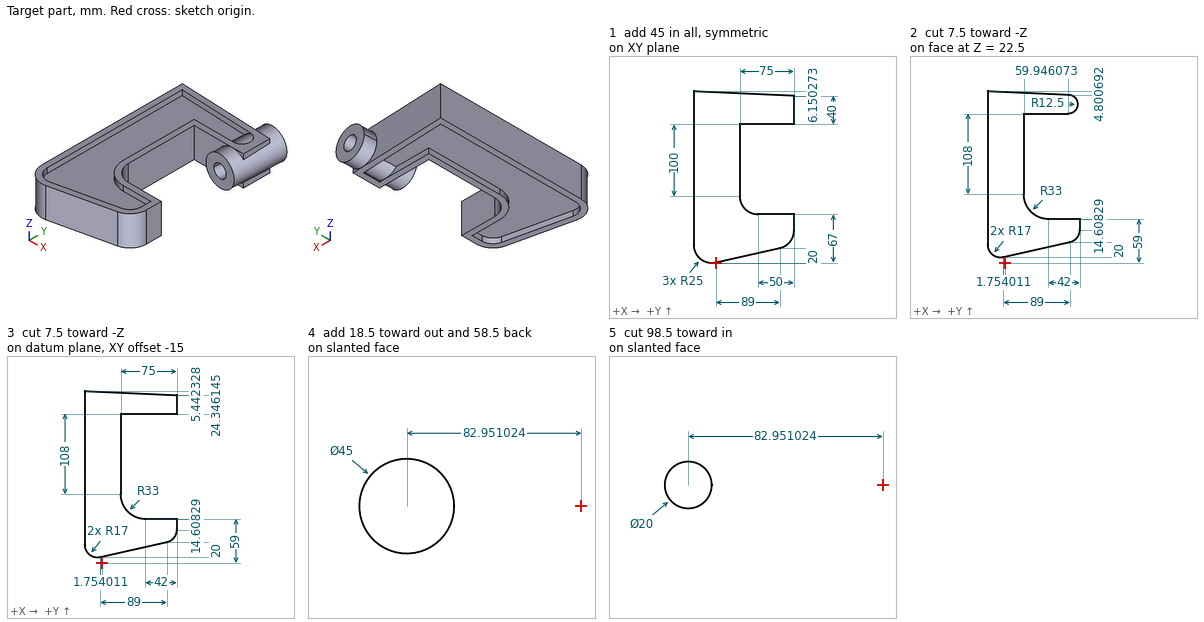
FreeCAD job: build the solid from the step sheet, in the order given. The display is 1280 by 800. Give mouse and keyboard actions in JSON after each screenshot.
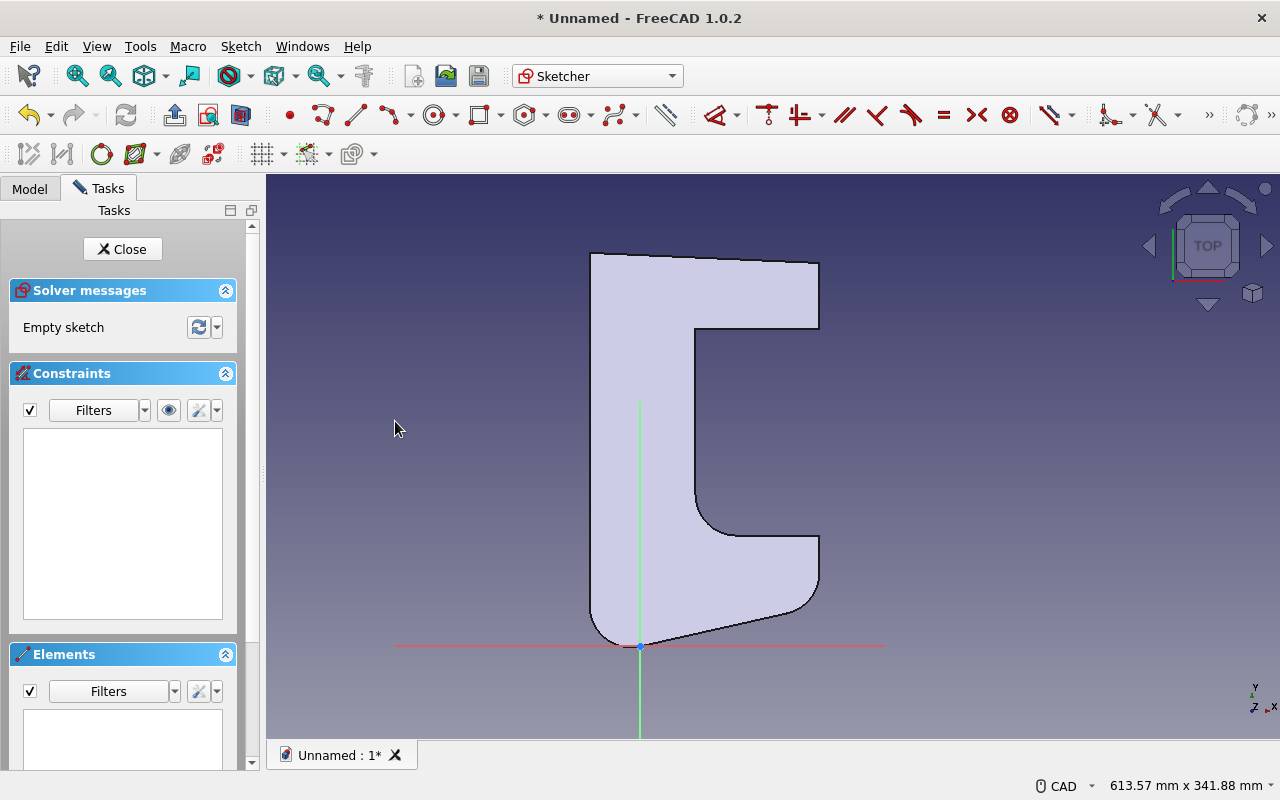
{"action": "left_click", "coordinate": [356, 116]}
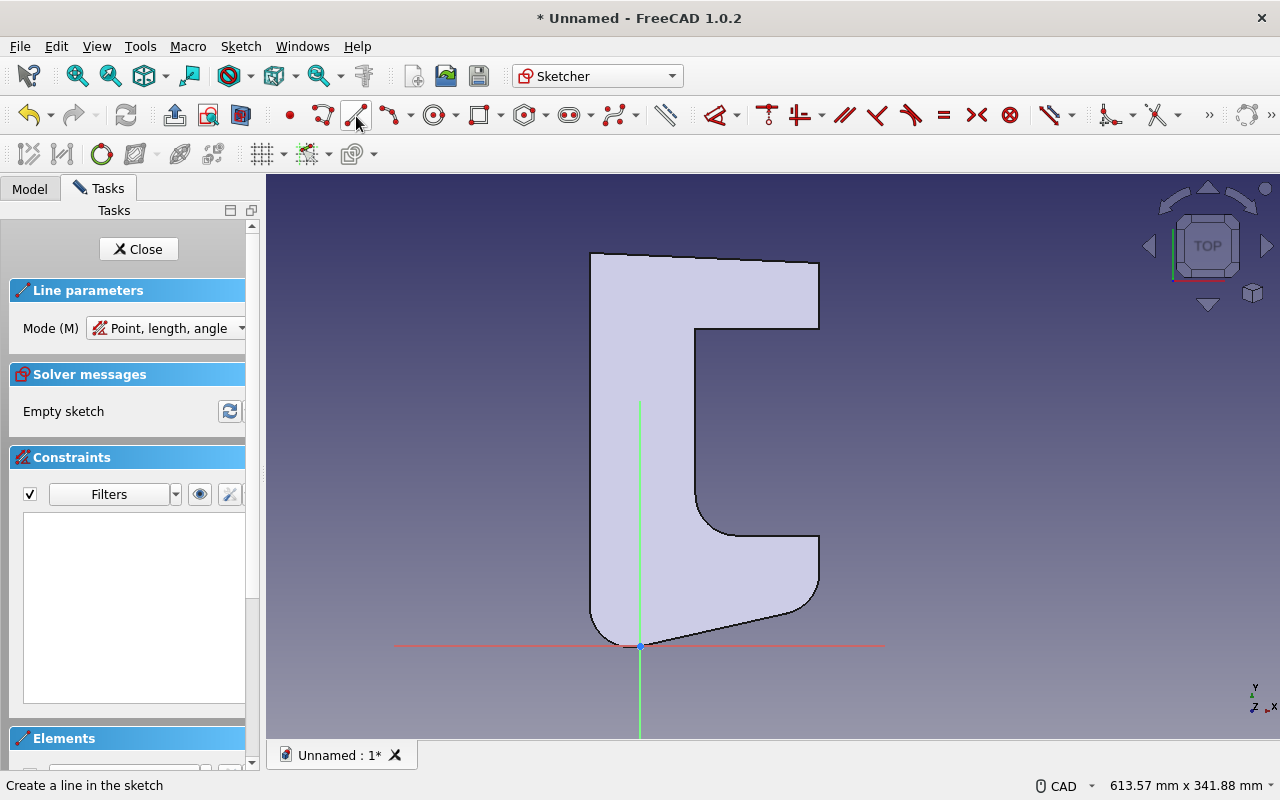
{"action": "scroll", "coordinate": [637, 634], "scroll_direction": "up", "scroll_amount": 9}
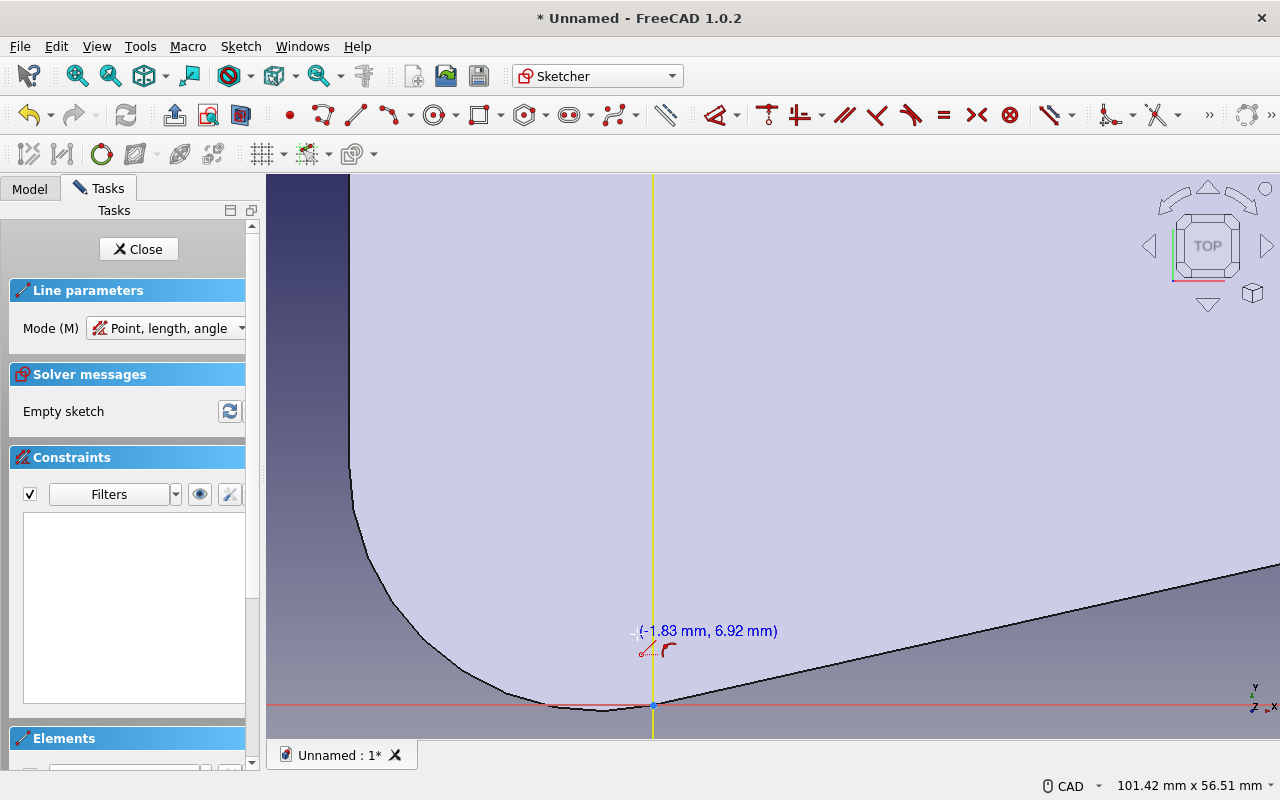
{"action": "left_click", "coordinate": [636, 627]}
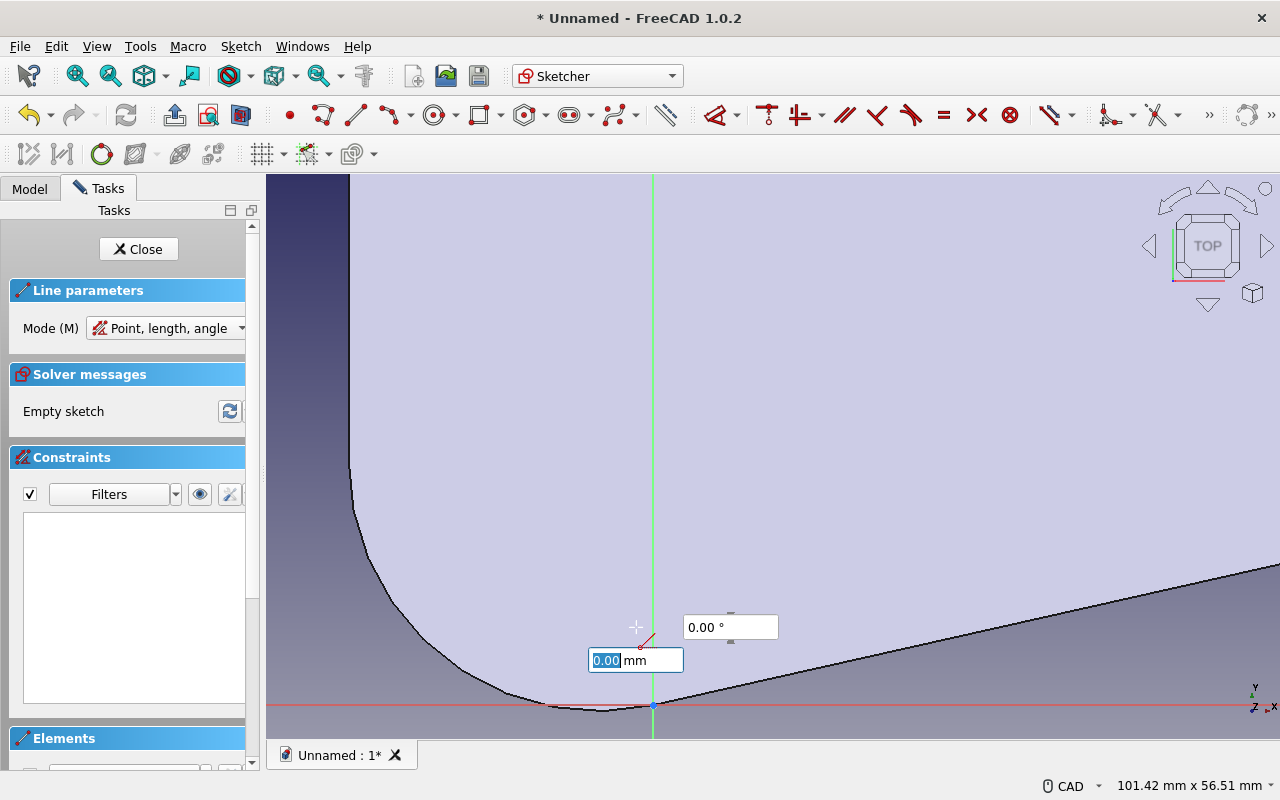
{"action": "scroll", "coordinate": [637, 635], "scroll_direction": "down", "scroll_amount": 9}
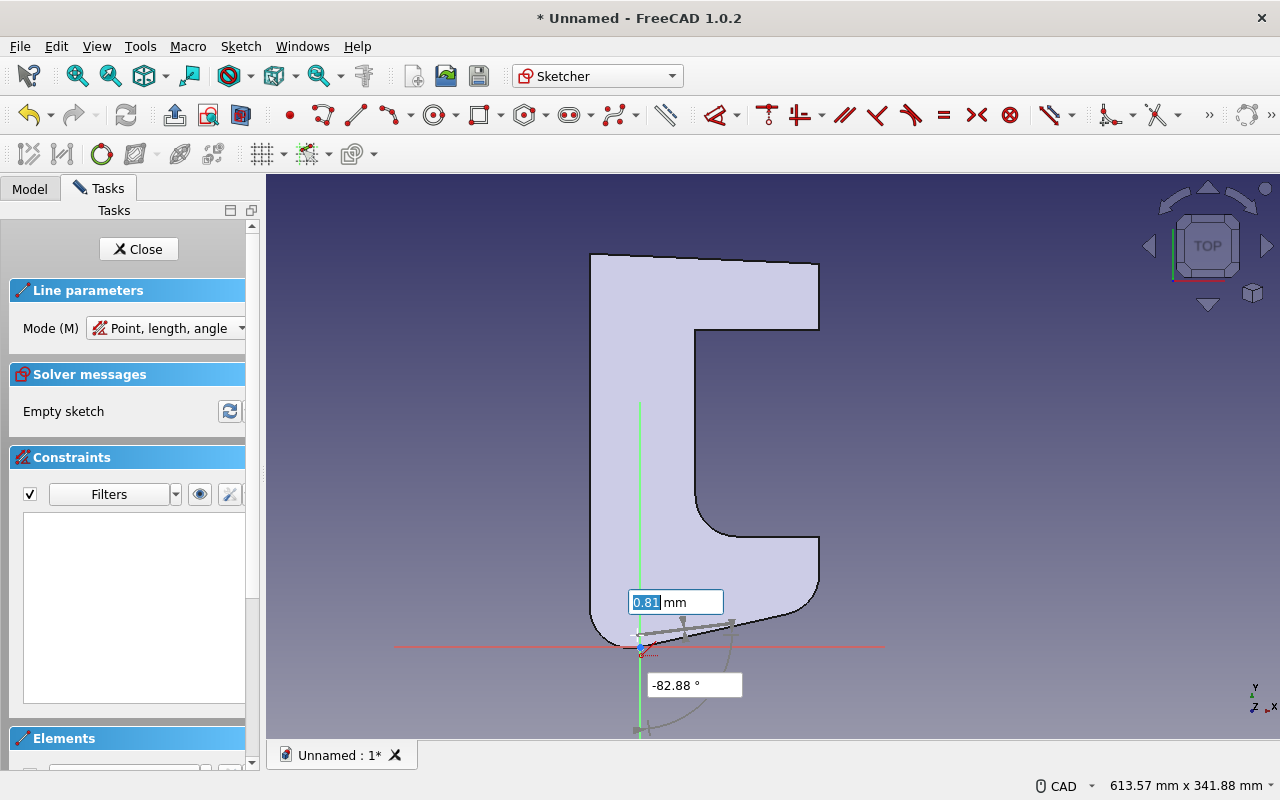
{"action": "left_click", "coordinate": [784, 601]}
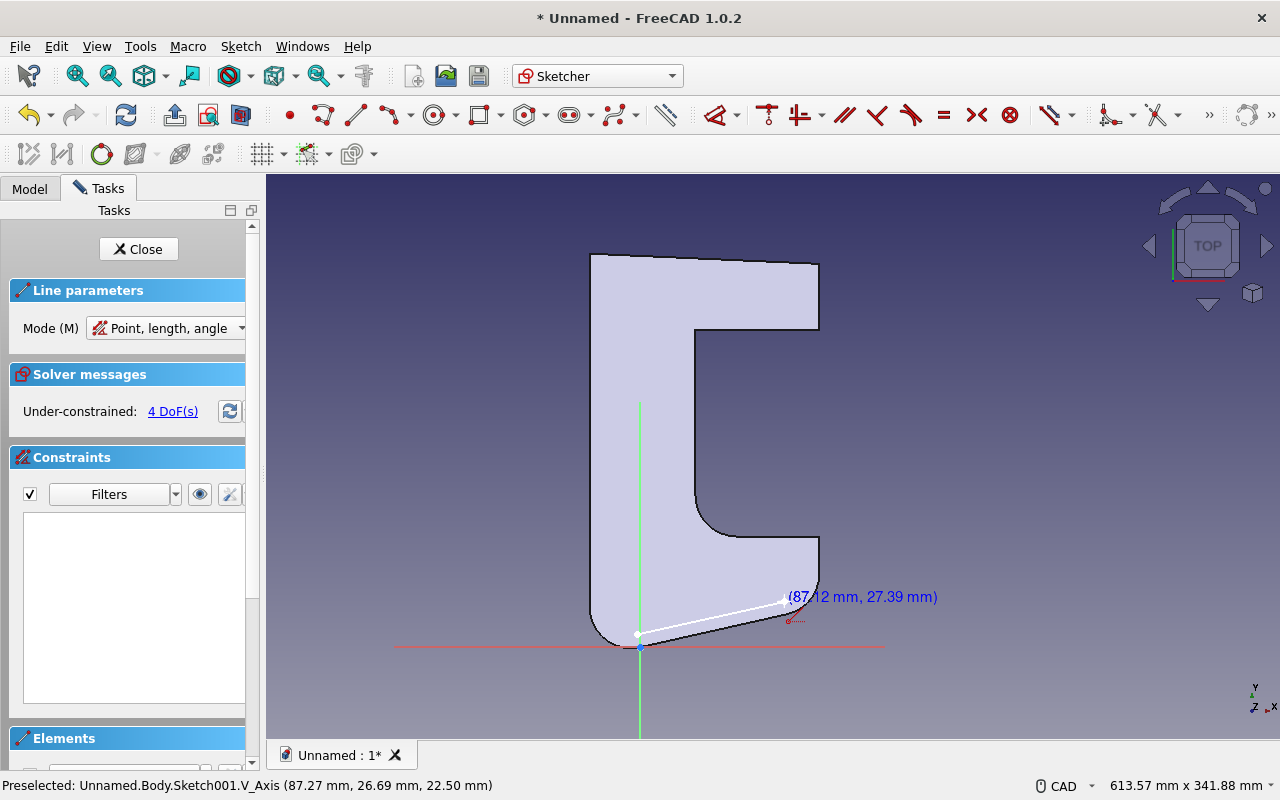
{"action": "left_click", "coordinate": [323, 116]}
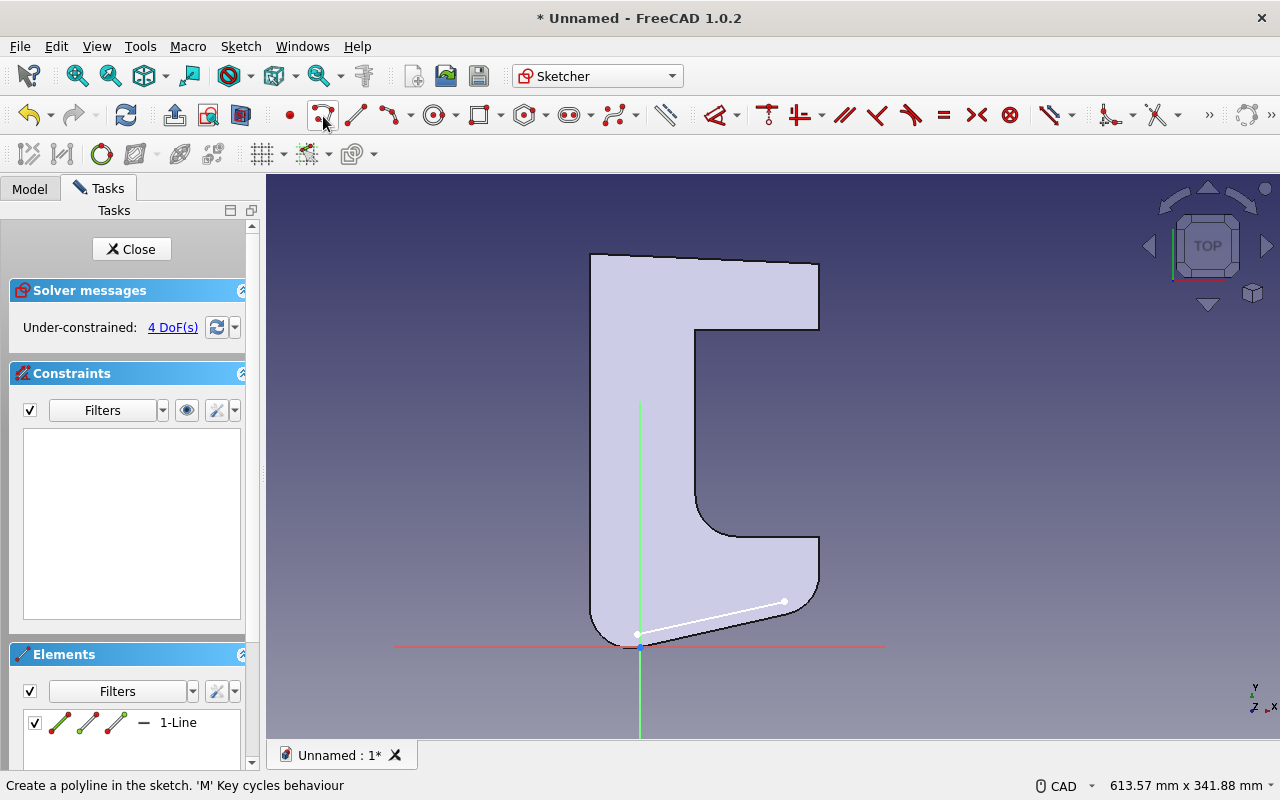
{"action": "left_click", "coordinate": [806, 574]}
{"action": "left_click", "coordinate": [806, 550]}
{"action": "left_click", "coordinate": [737, 550]}
{"action": "right_click", "coordinate": [737, 550]}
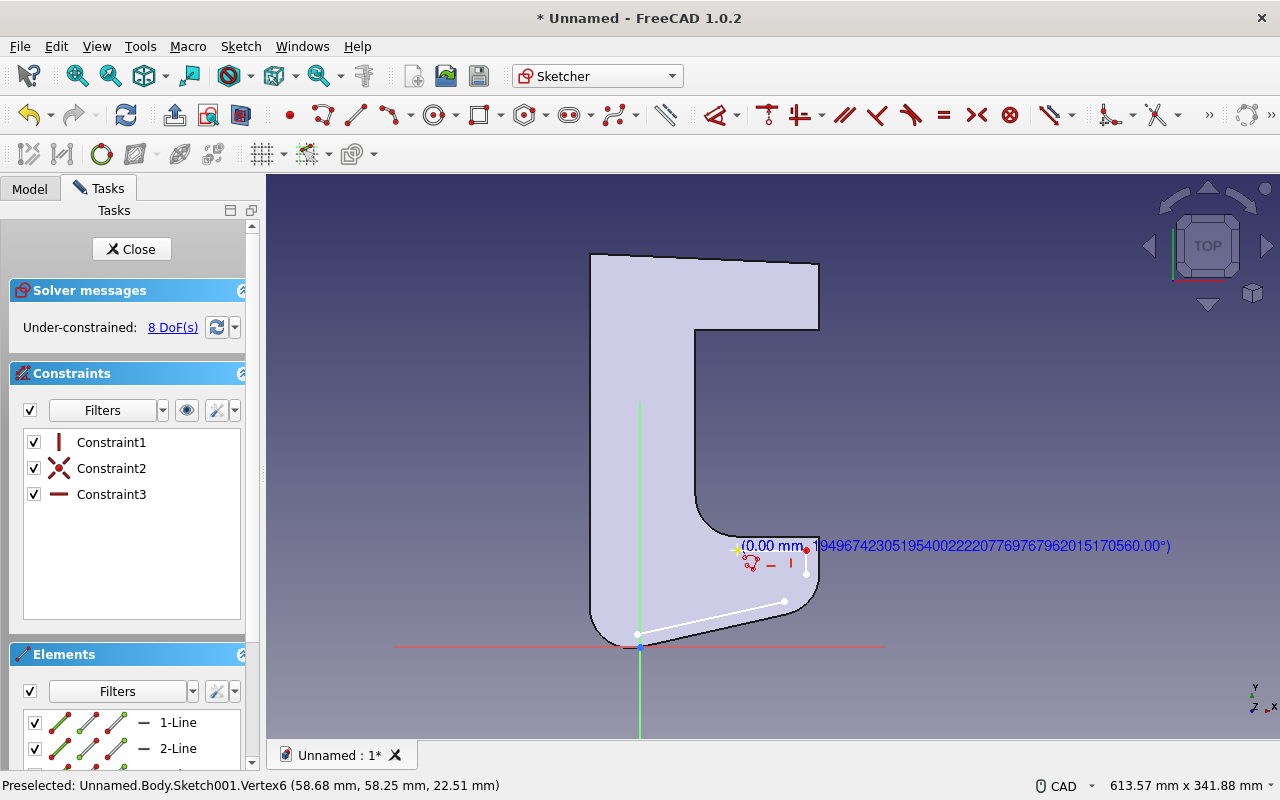
{"action": "left_click", "coordinate": [682, 495]}
{"action": "left_click", "coordinate": [682, 317]}
{"action": "left_click", "coordinate": [781, 317]}
{"action": "right_click", "coordinate": [781, 317]}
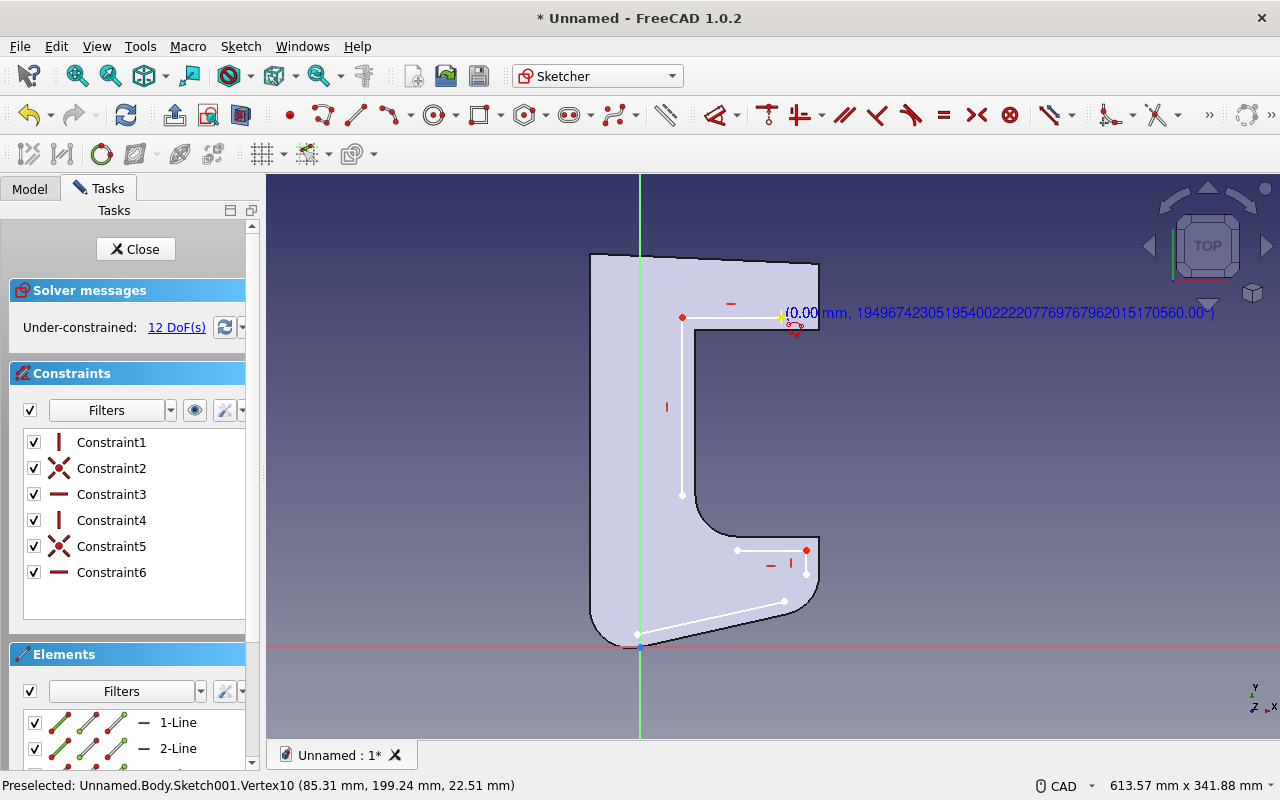
{"action": "left_click", "coordinate": [782, 275]}
{"action": "left_click", "coordinate": [603, 265]}
{"action": "left_click", "coordinate": [603, 607]}
{"action": "right_click", "coordinate": [603, 607]}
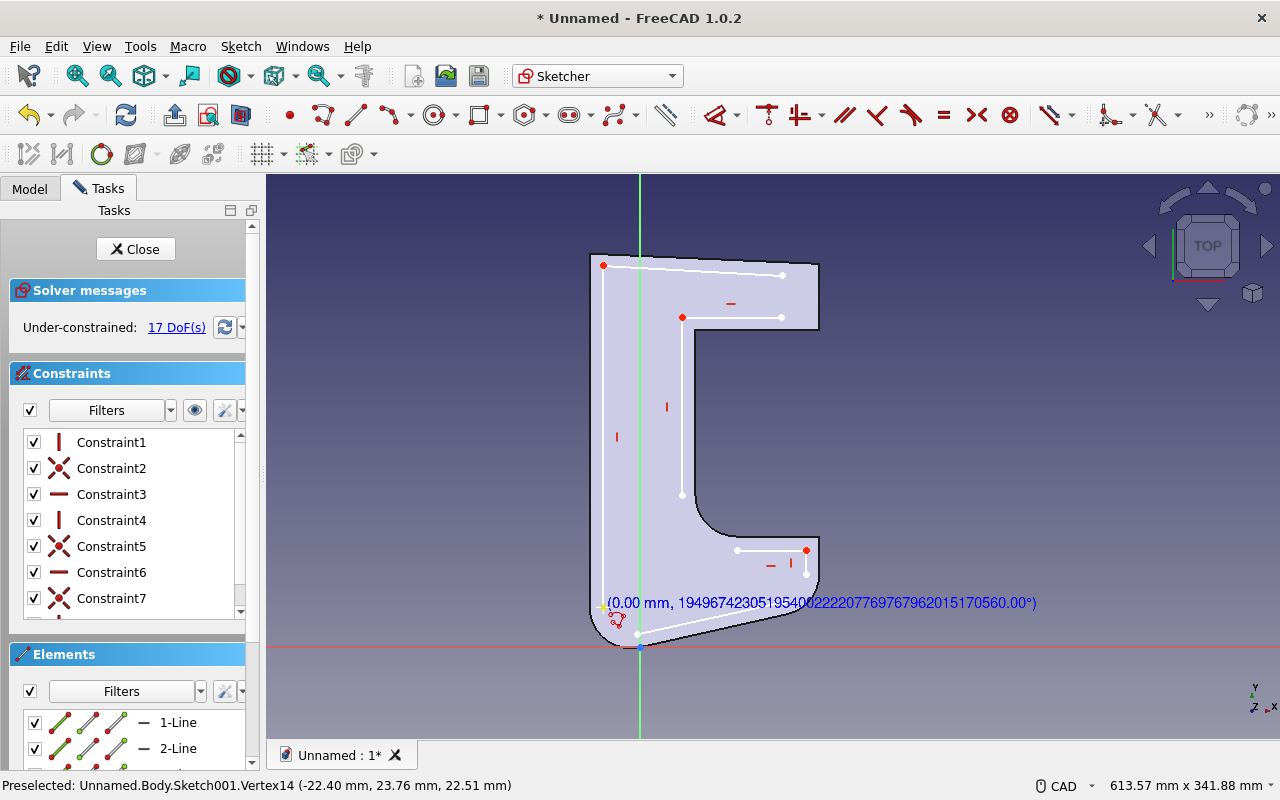
{"action": "left_click", "coordinate": [388, 116]}